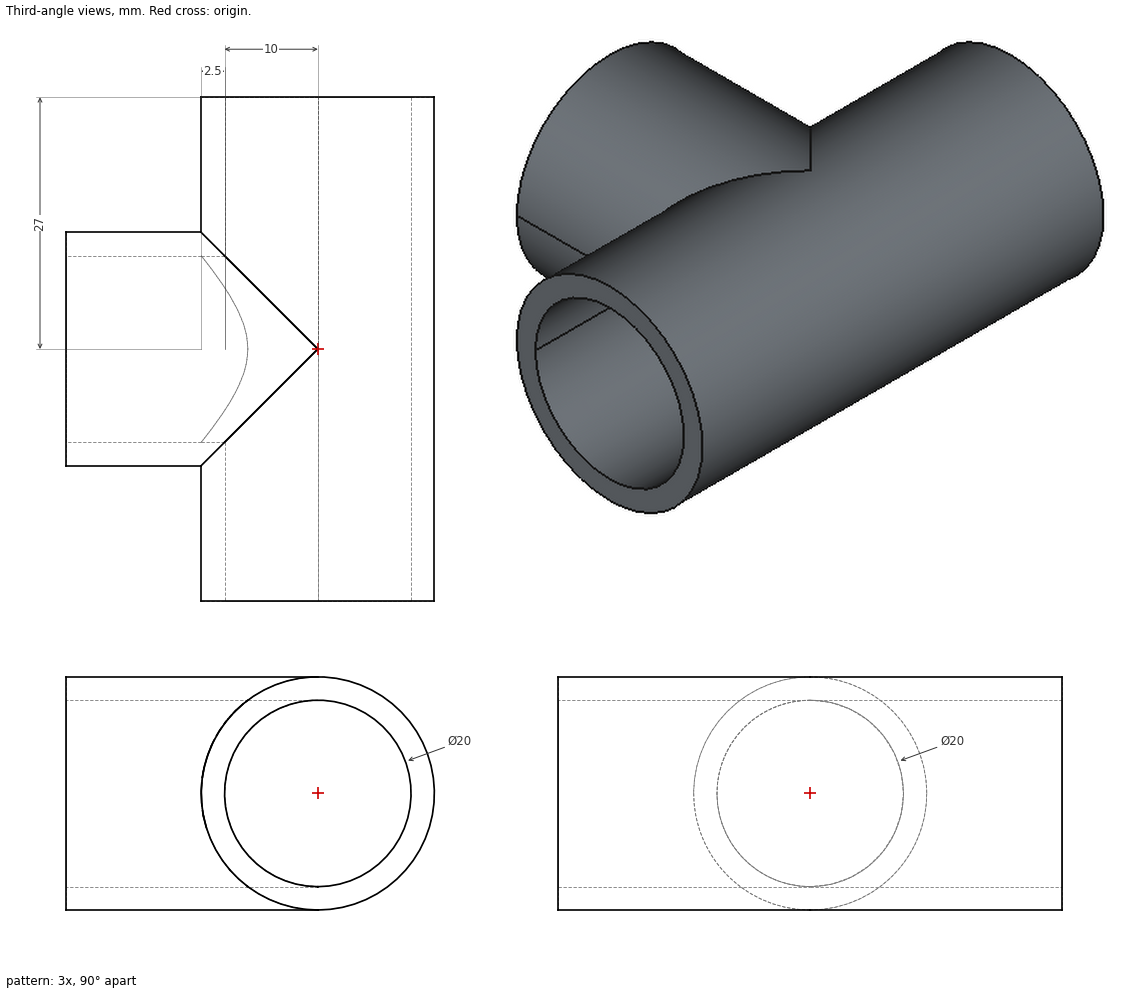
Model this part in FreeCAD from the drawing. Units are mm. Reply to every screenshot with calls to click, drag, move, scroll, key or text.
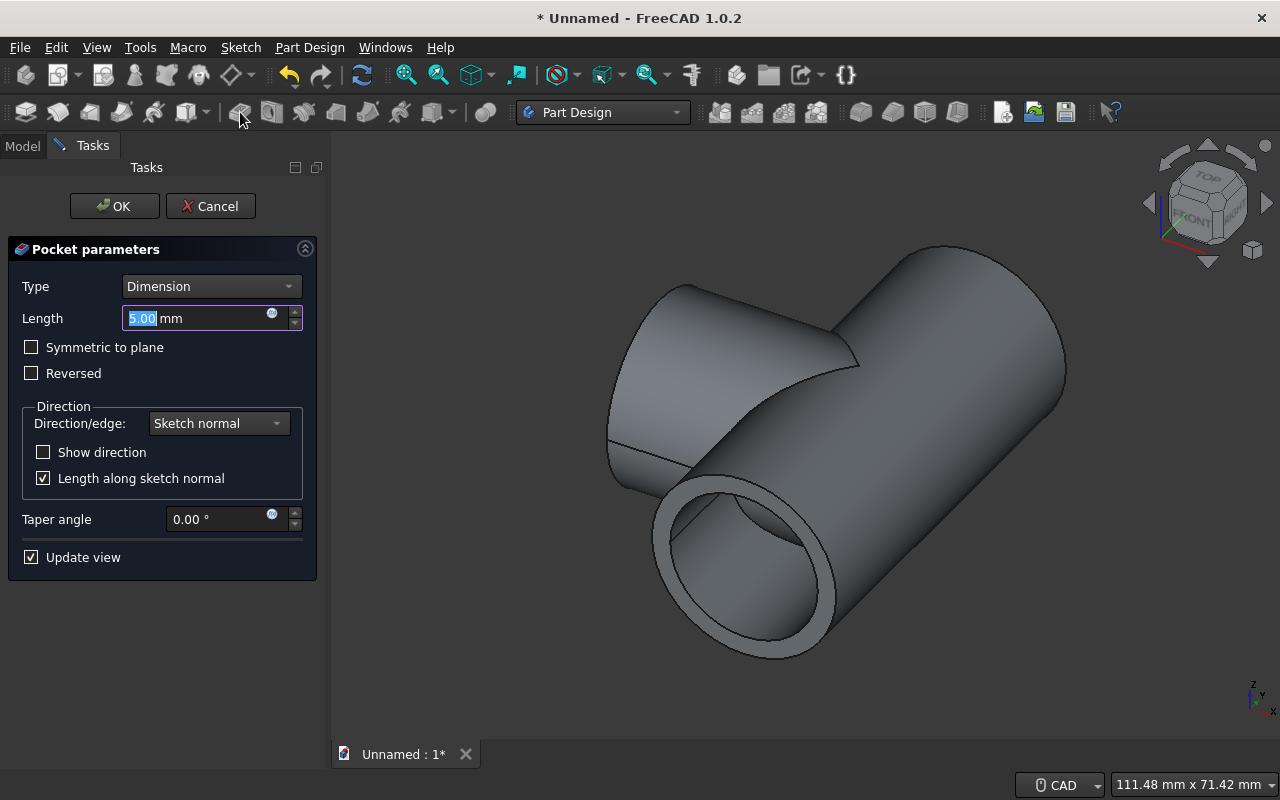
click(212, 286)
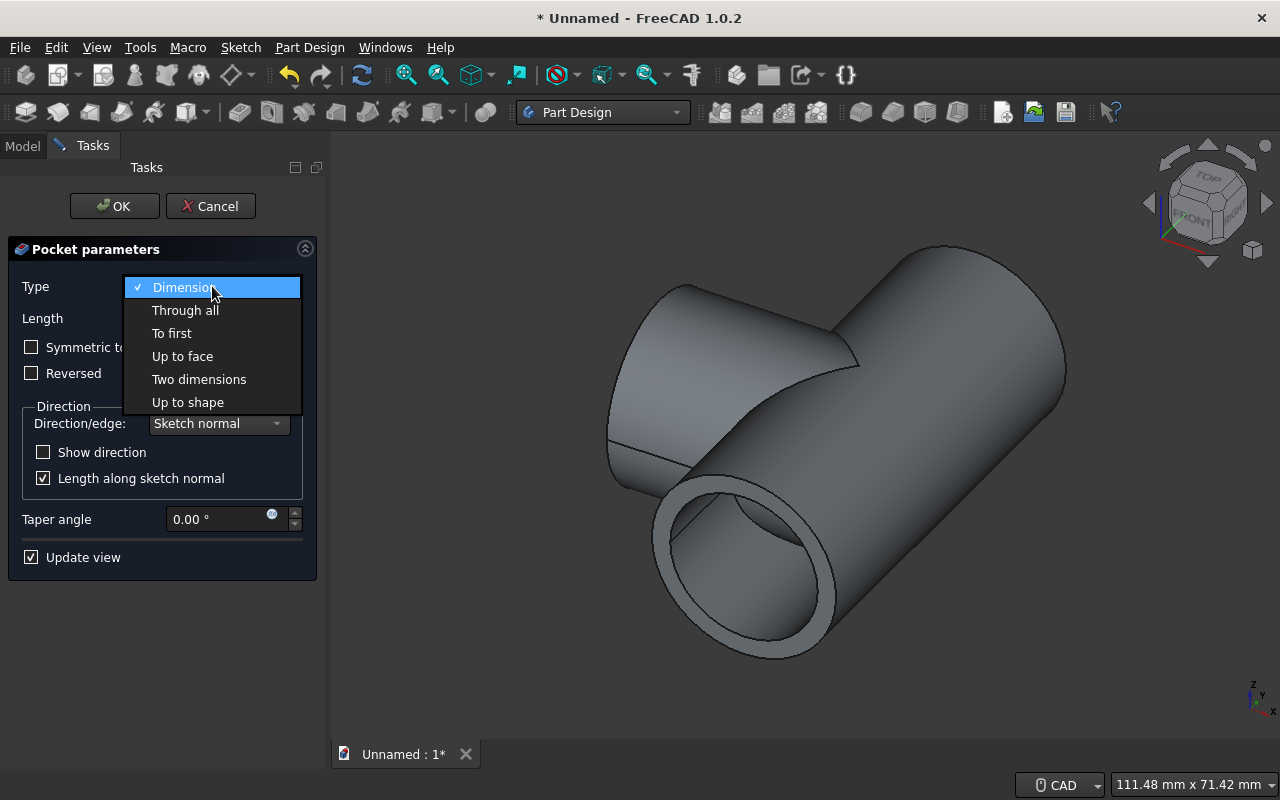
click(212, 310)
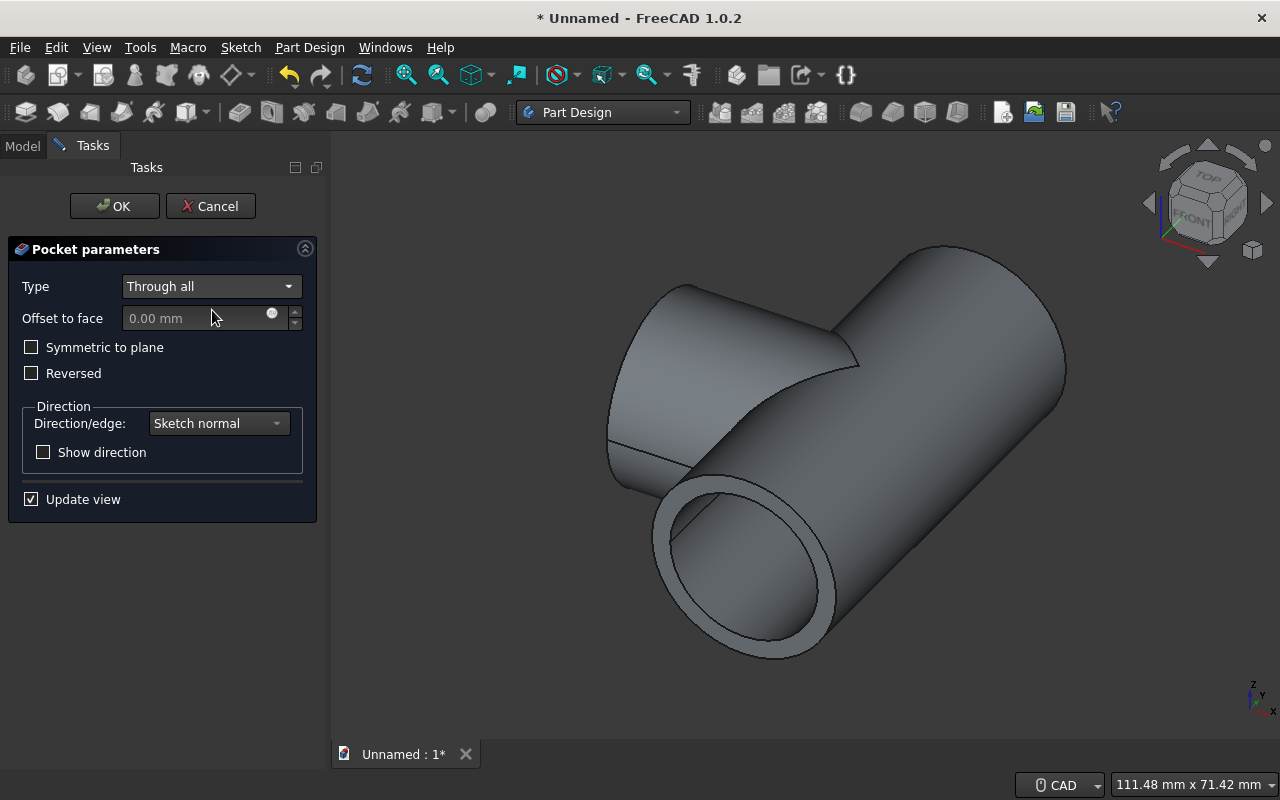
click(115, 206)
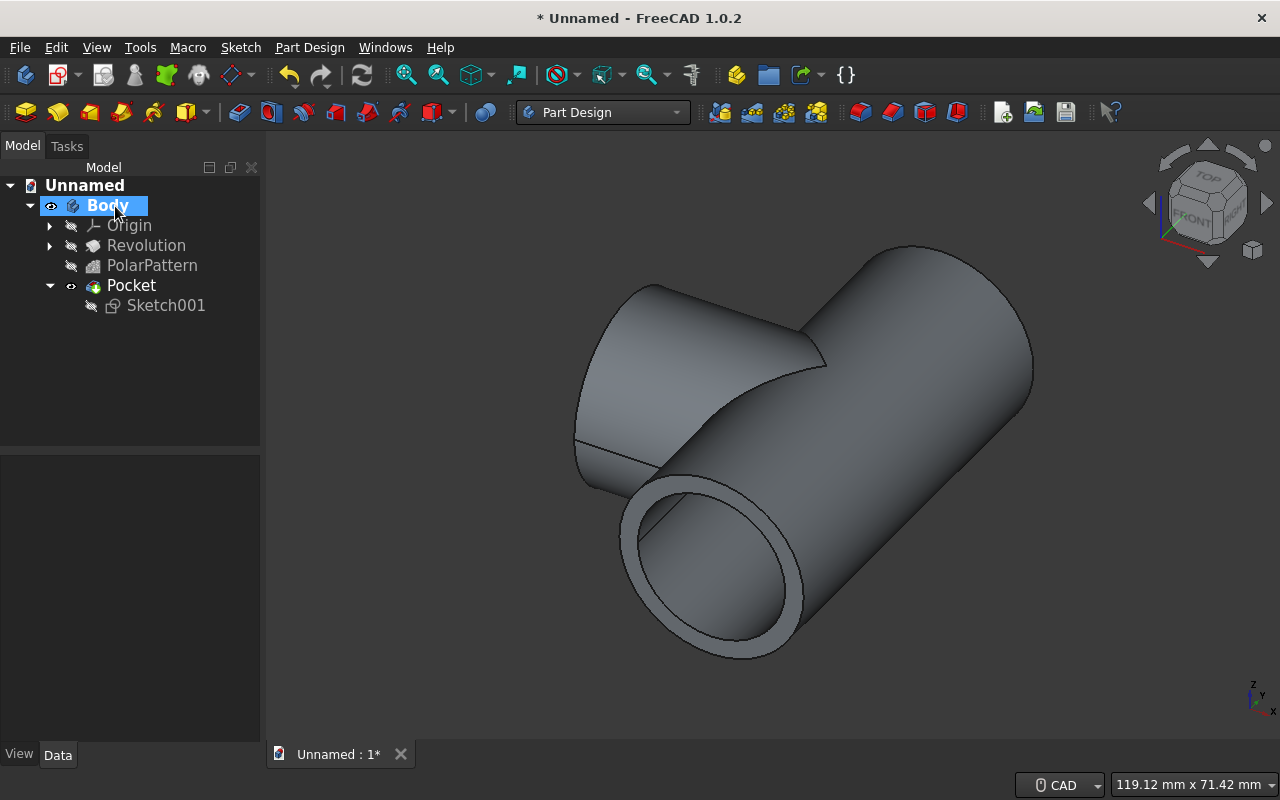
click(58, 76)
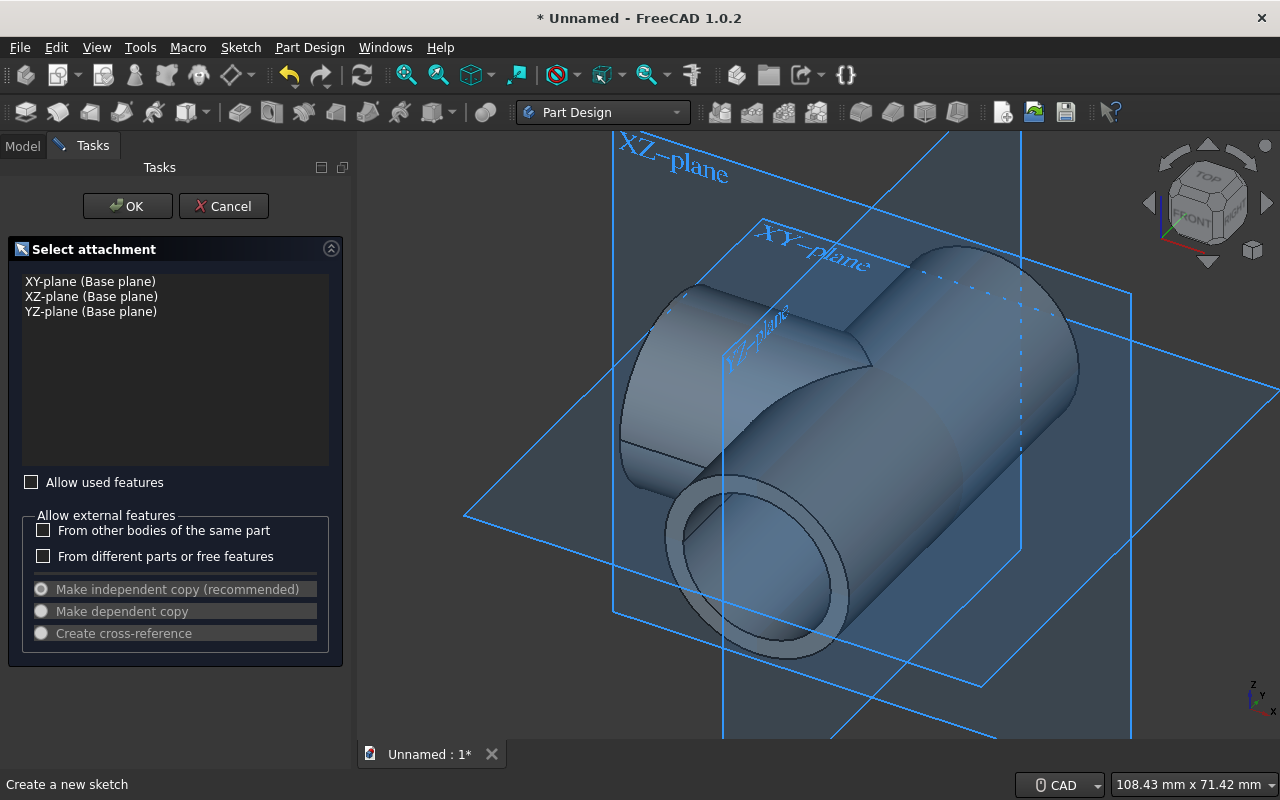
click(82, 312)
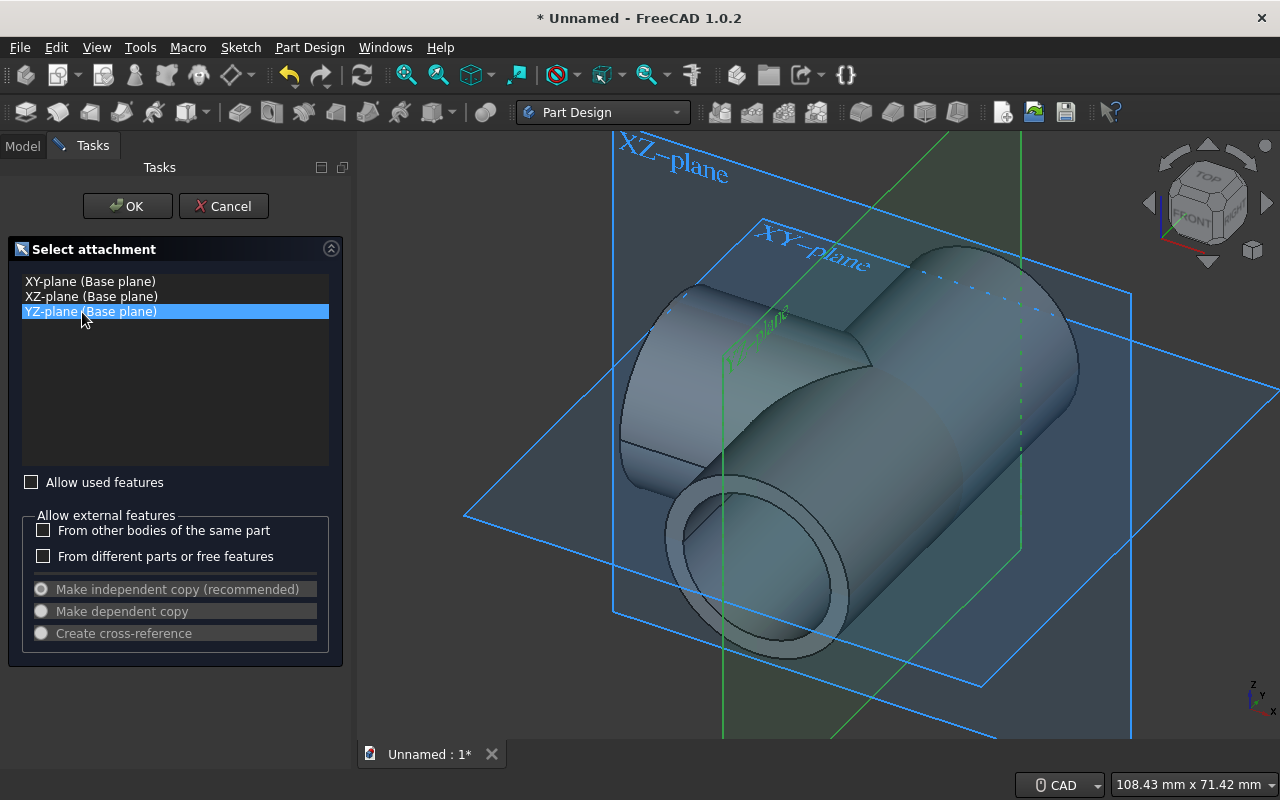
click(128, 206)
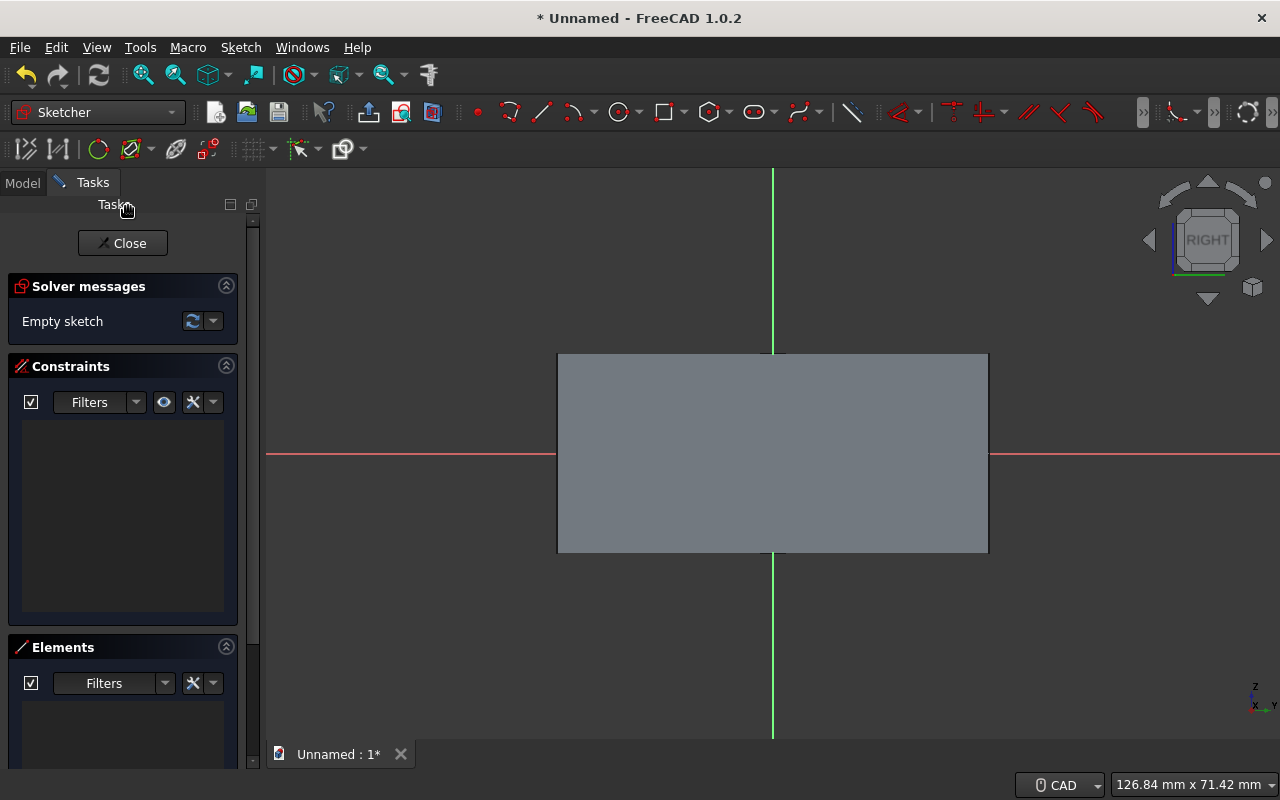
key(q)
key(s)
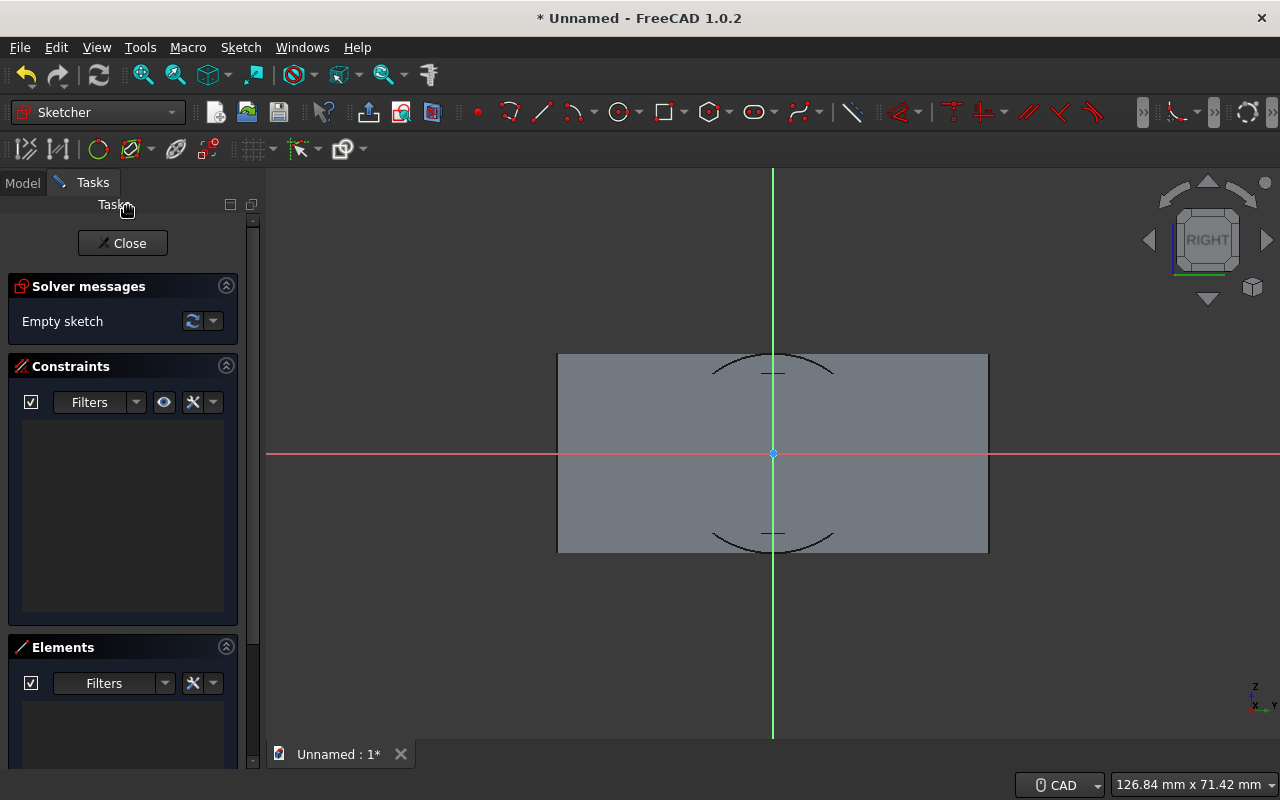
scroll(829, 454, up, 4)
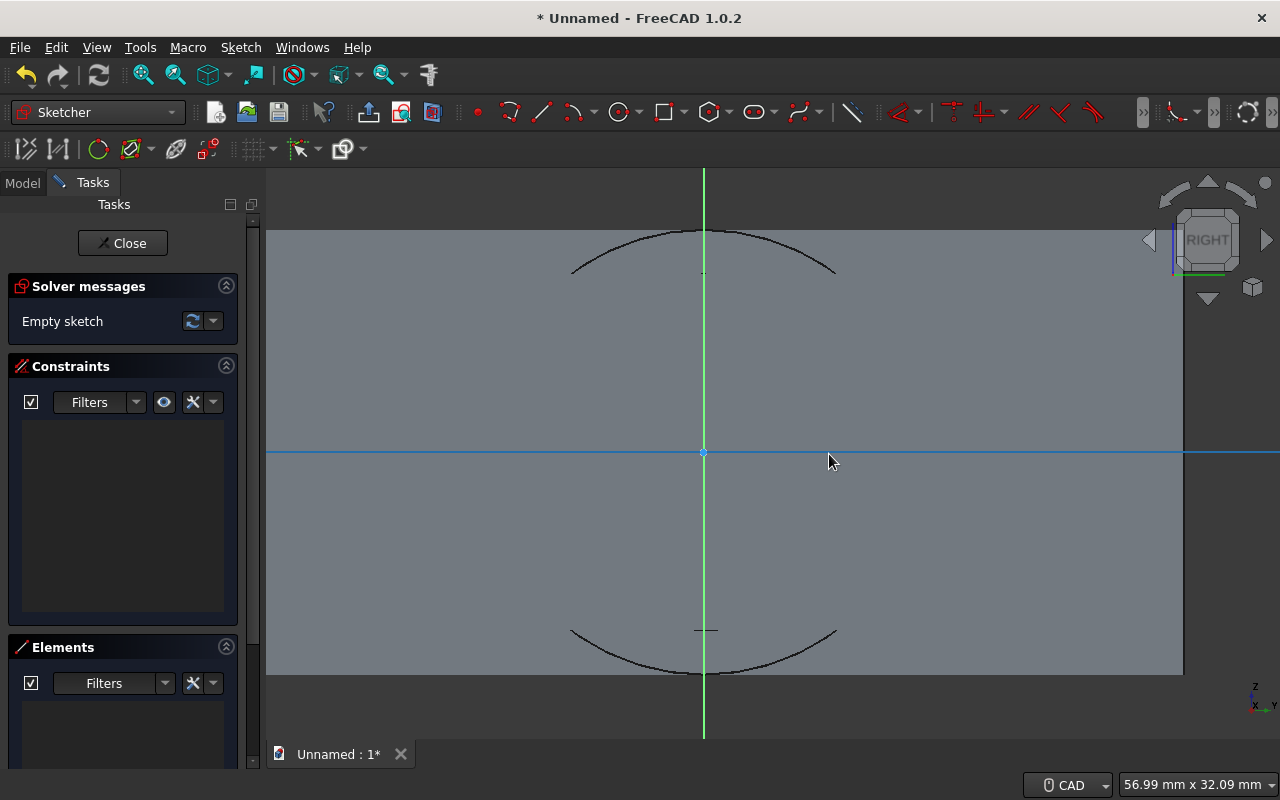
key(g)
key(c)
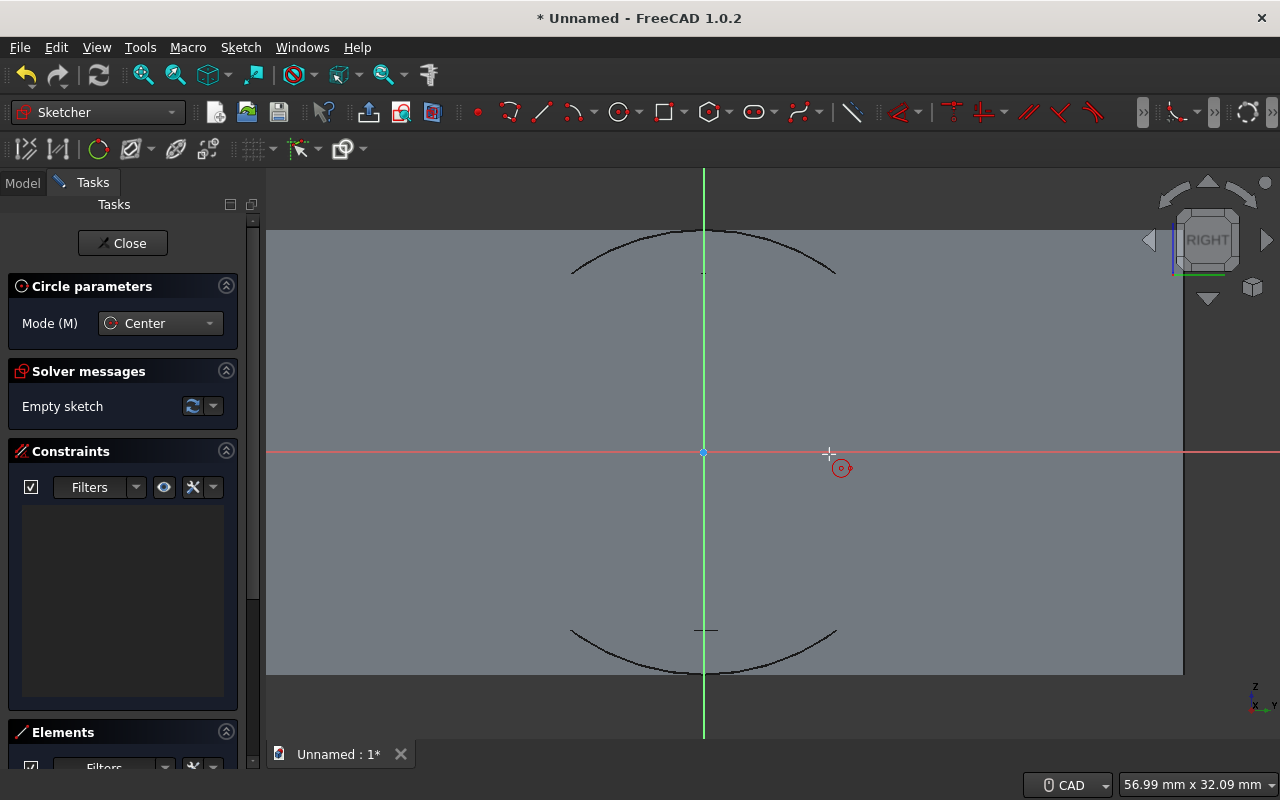
click(704, 452)
move(829, 326)